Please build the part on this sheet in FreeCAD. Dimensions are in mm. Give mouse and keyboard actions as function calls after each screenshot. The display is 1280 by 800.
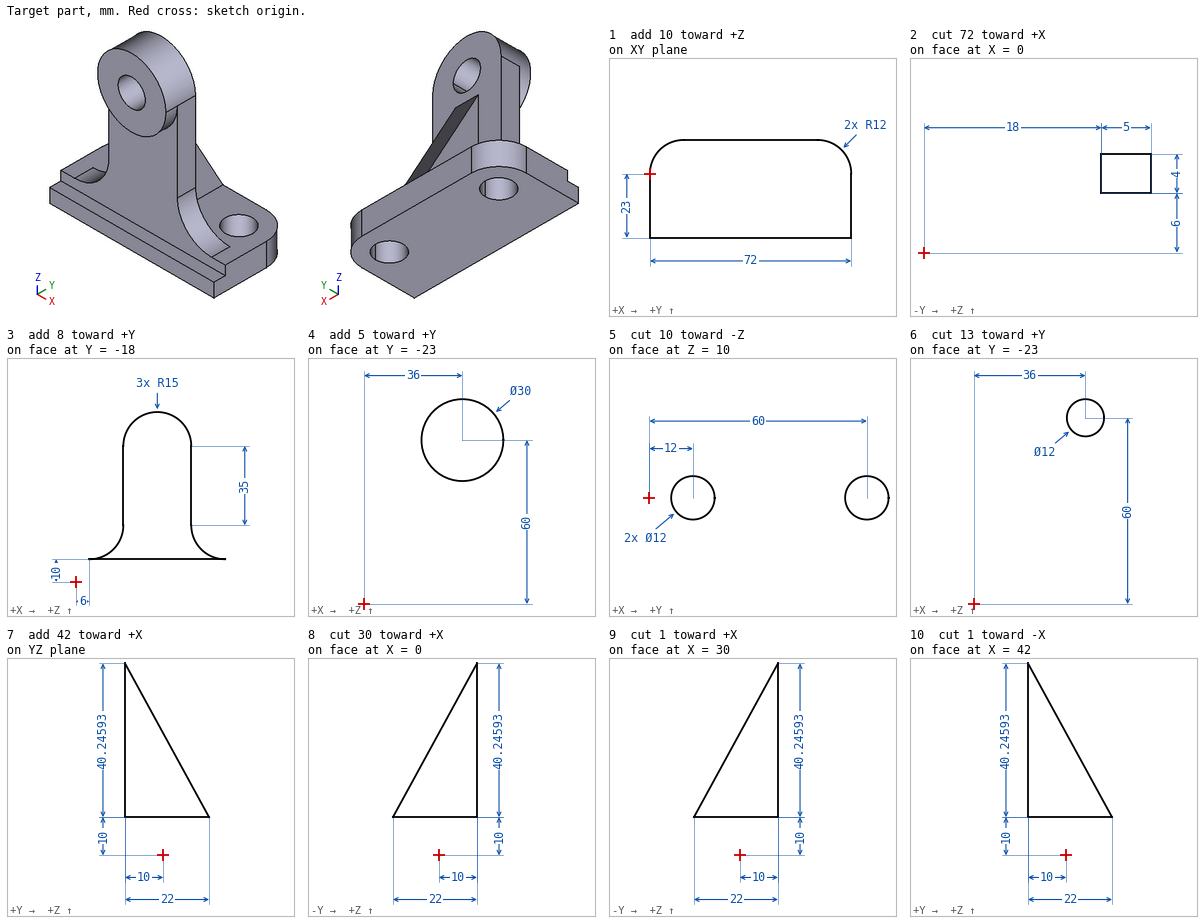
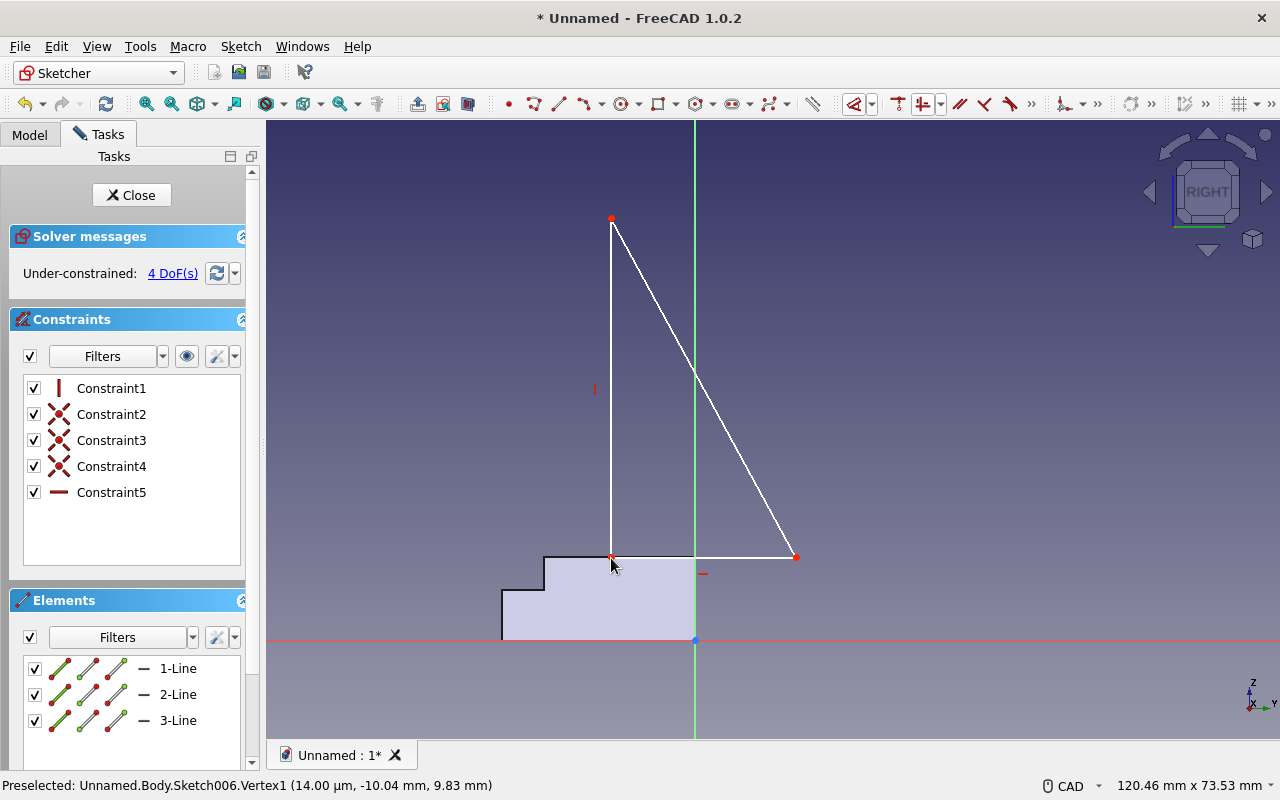
click(741, 558)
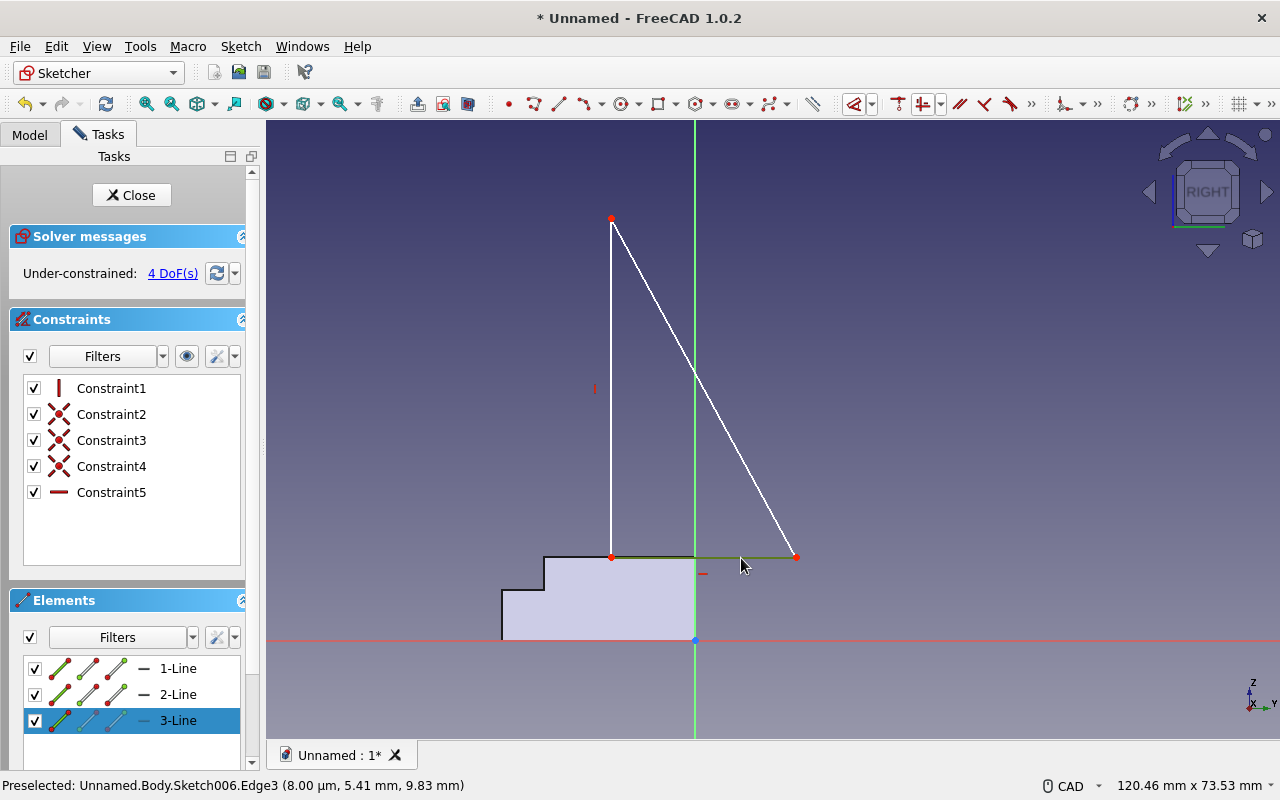
click(872, 104)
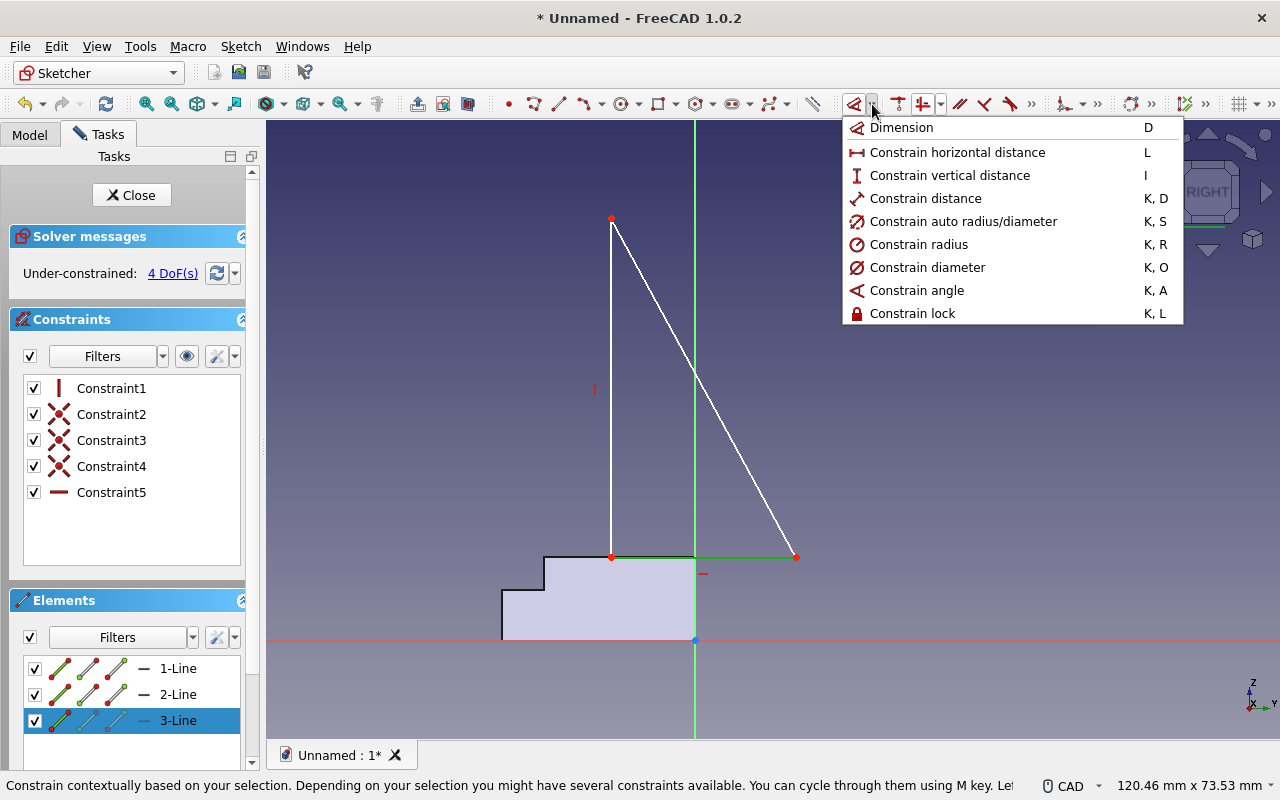
click(1013, 152)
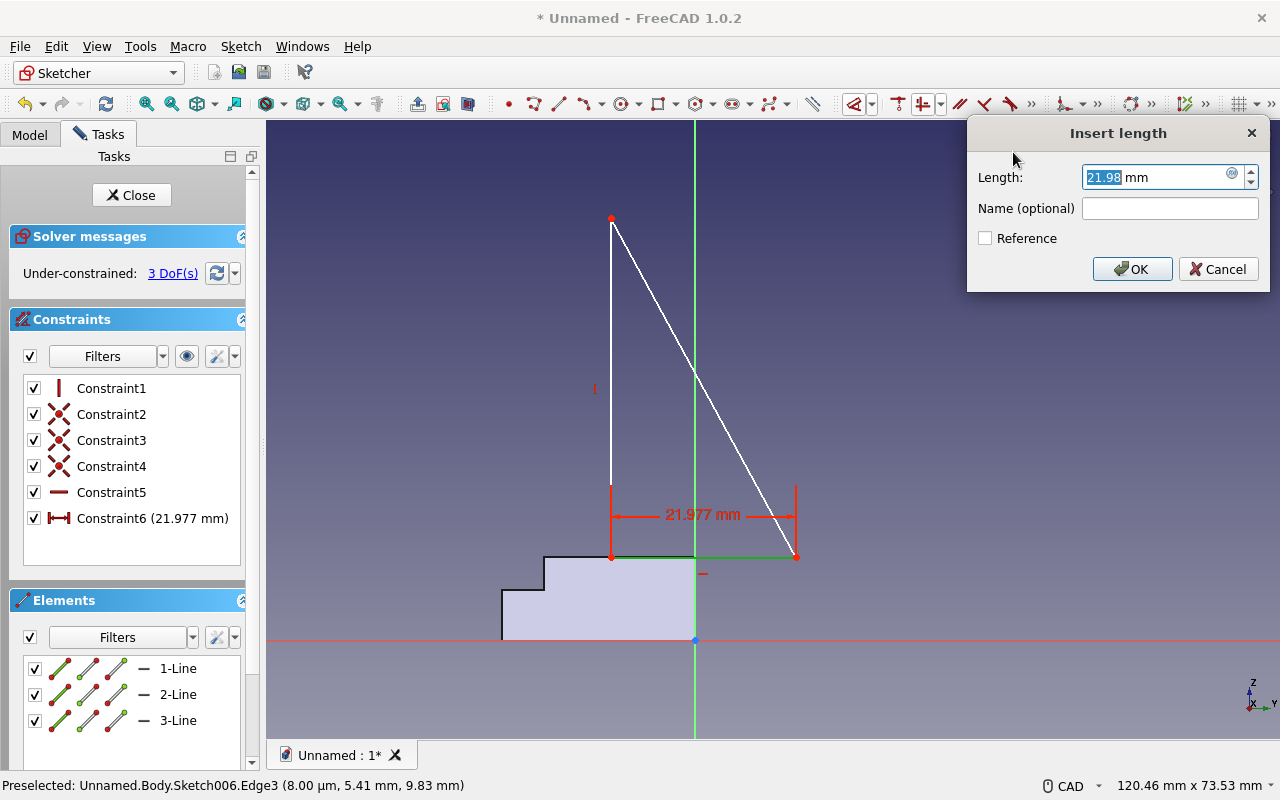
text(22)
key(Return)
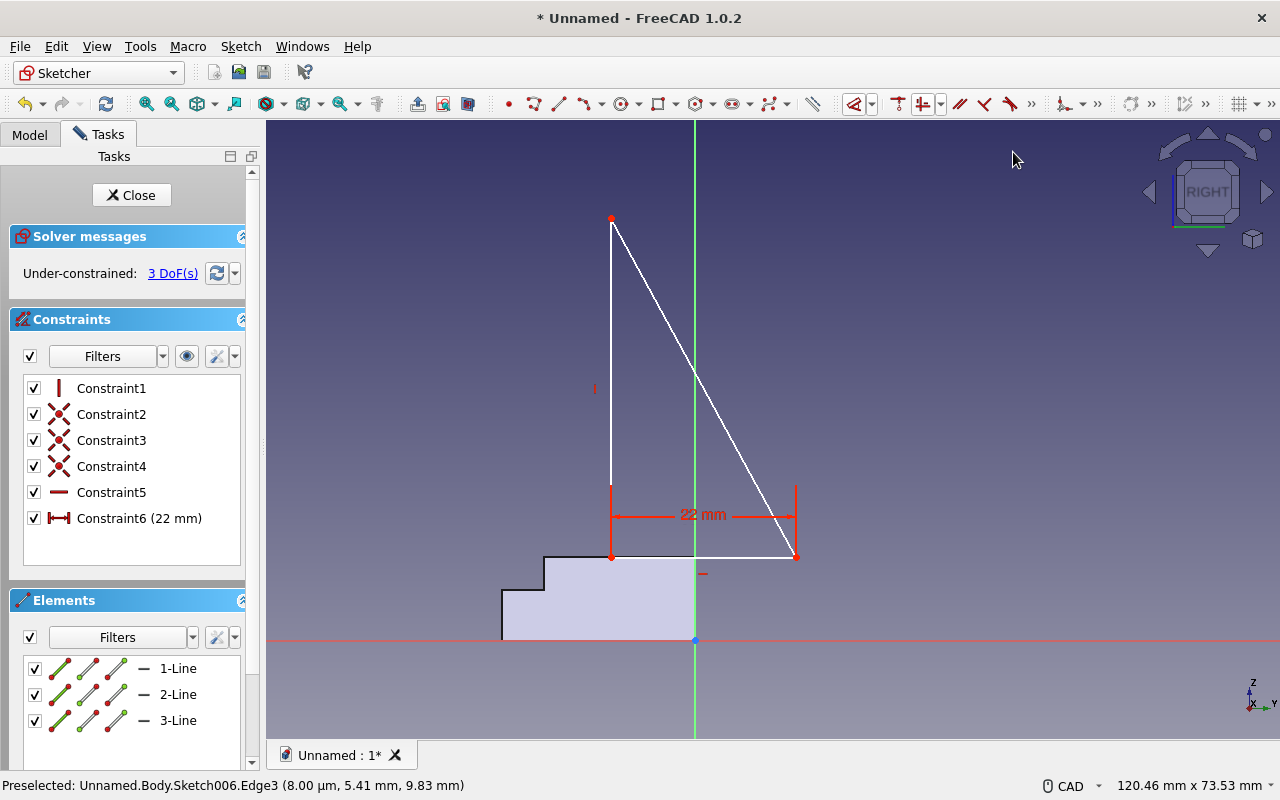
click(611, 558)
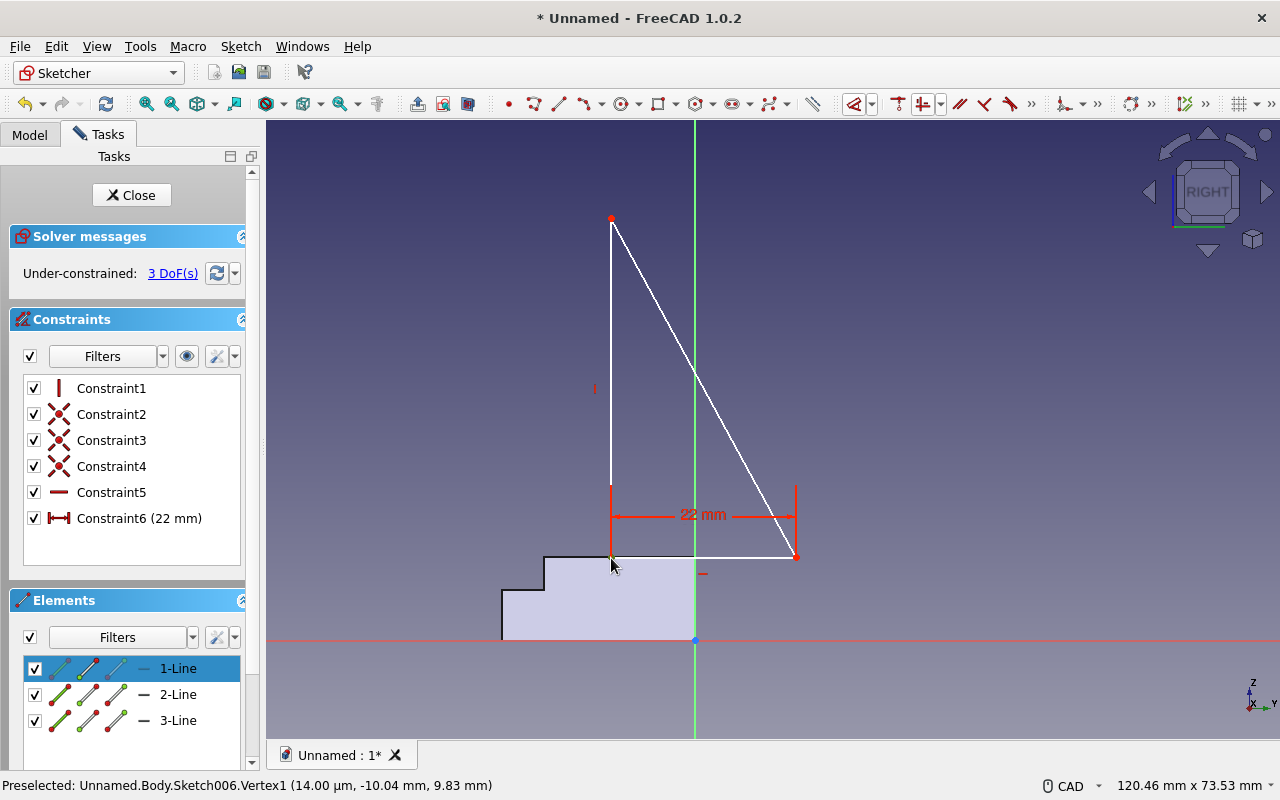
click(872, 104)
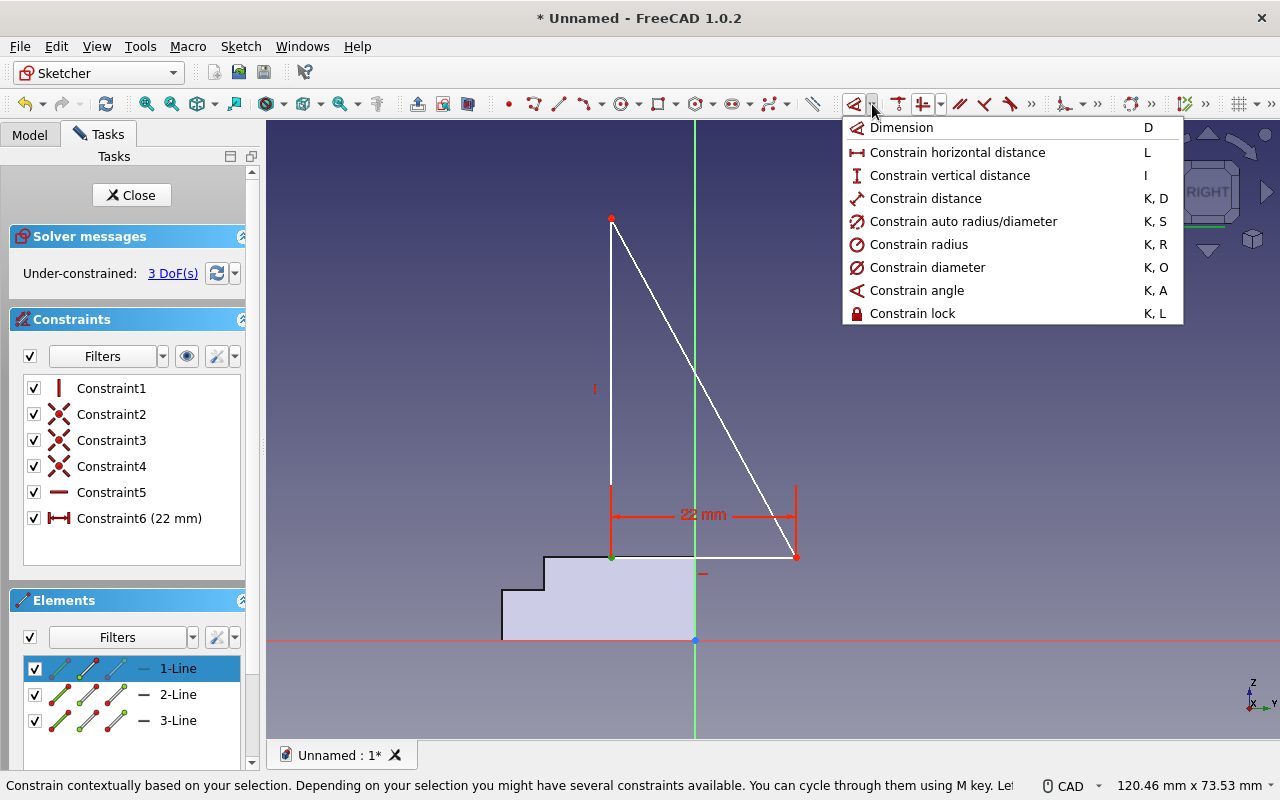
click(1013, 152)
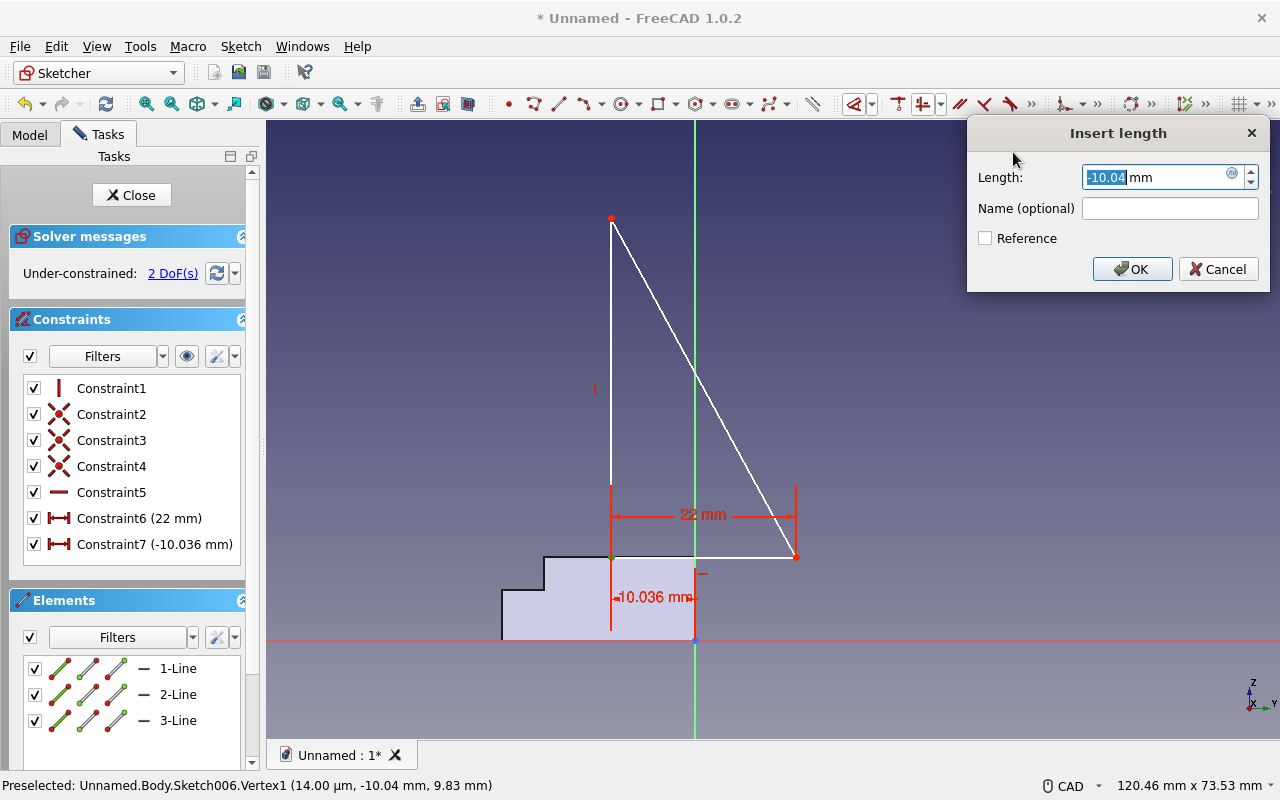
text(-10)
key(Return)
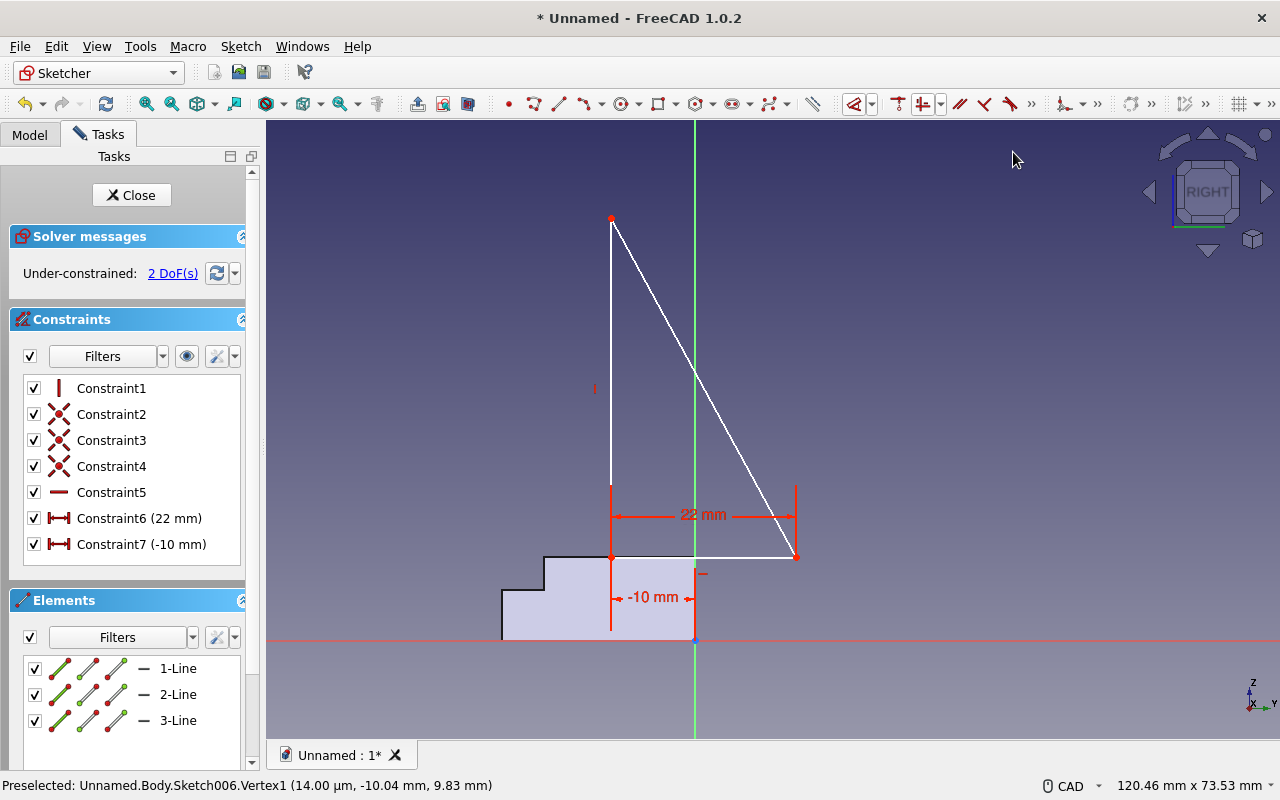
click(611, 558)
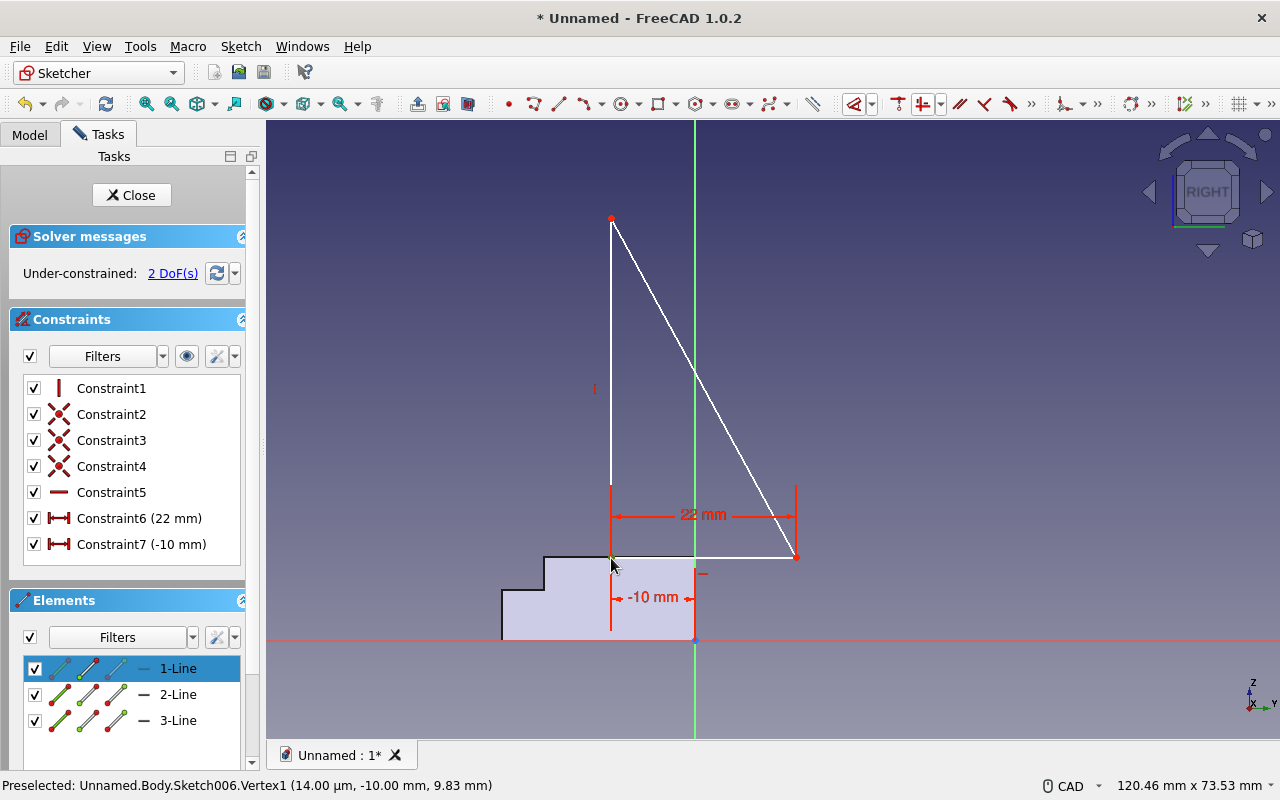
key(i)